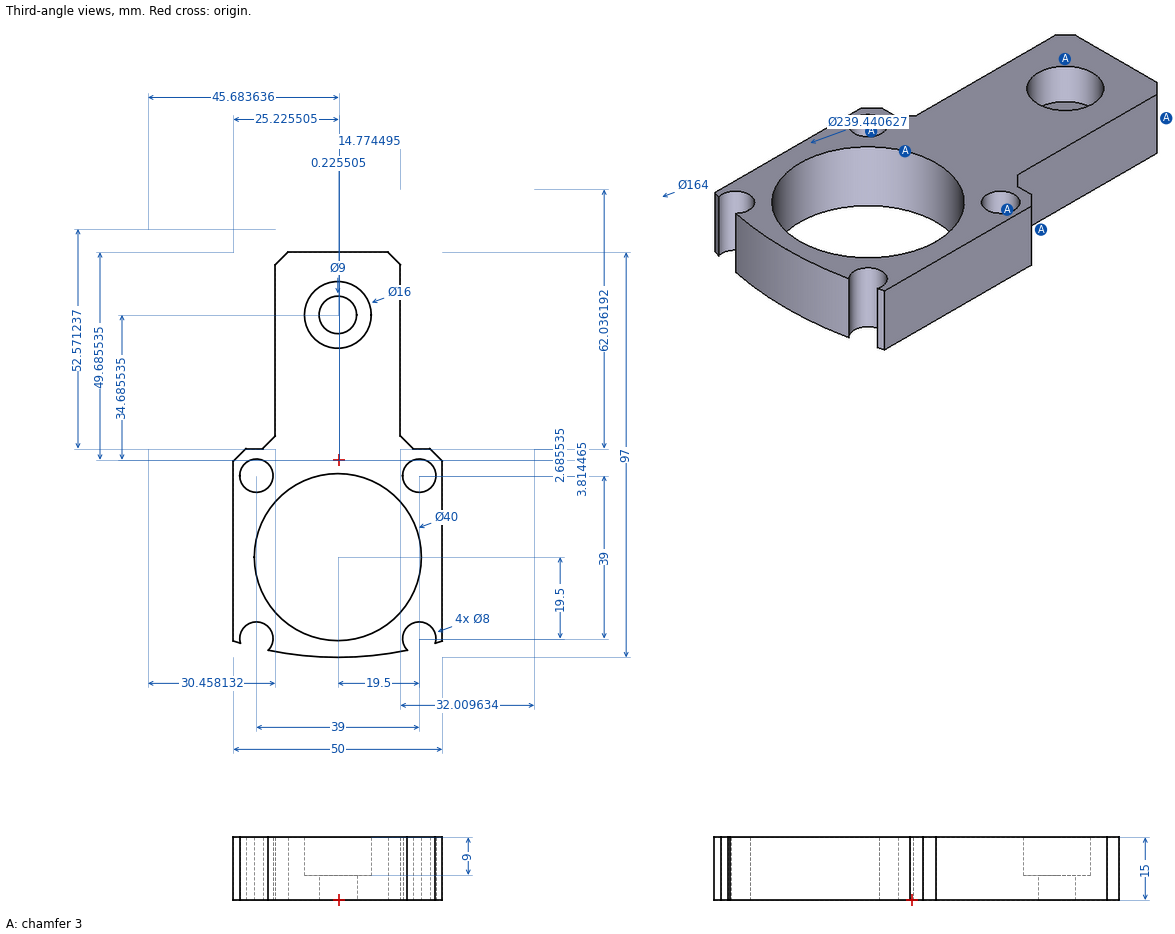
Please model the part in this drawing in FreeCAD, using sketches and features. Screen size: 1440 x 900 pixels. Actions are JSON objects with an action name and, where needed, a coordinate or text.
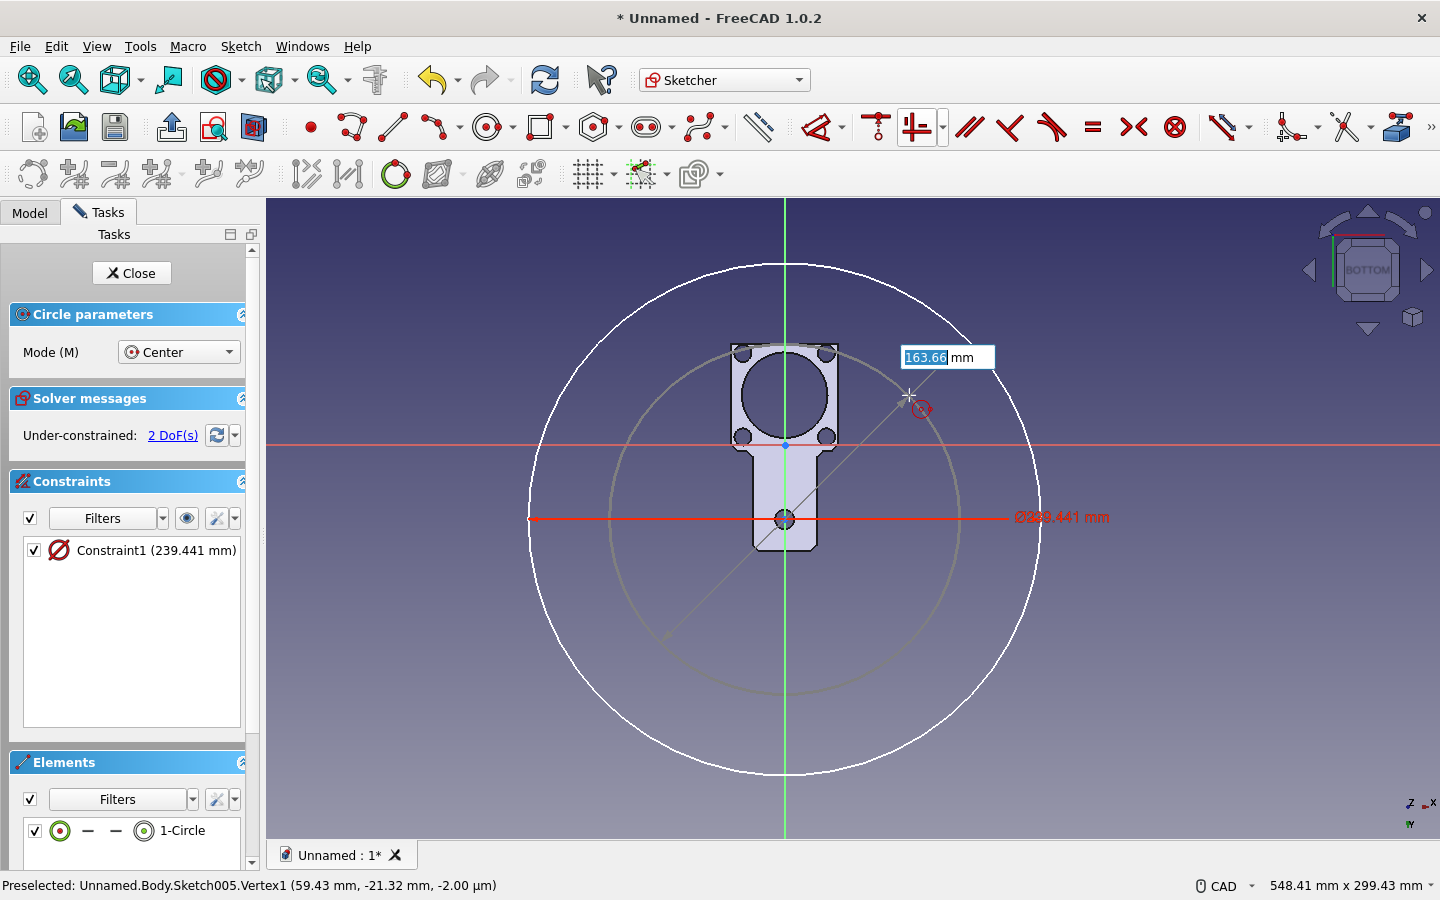
{"action": "type", "text": "164"}
{"action": "key", "text": "Return"}
{"action": "key", "text": "Escape"}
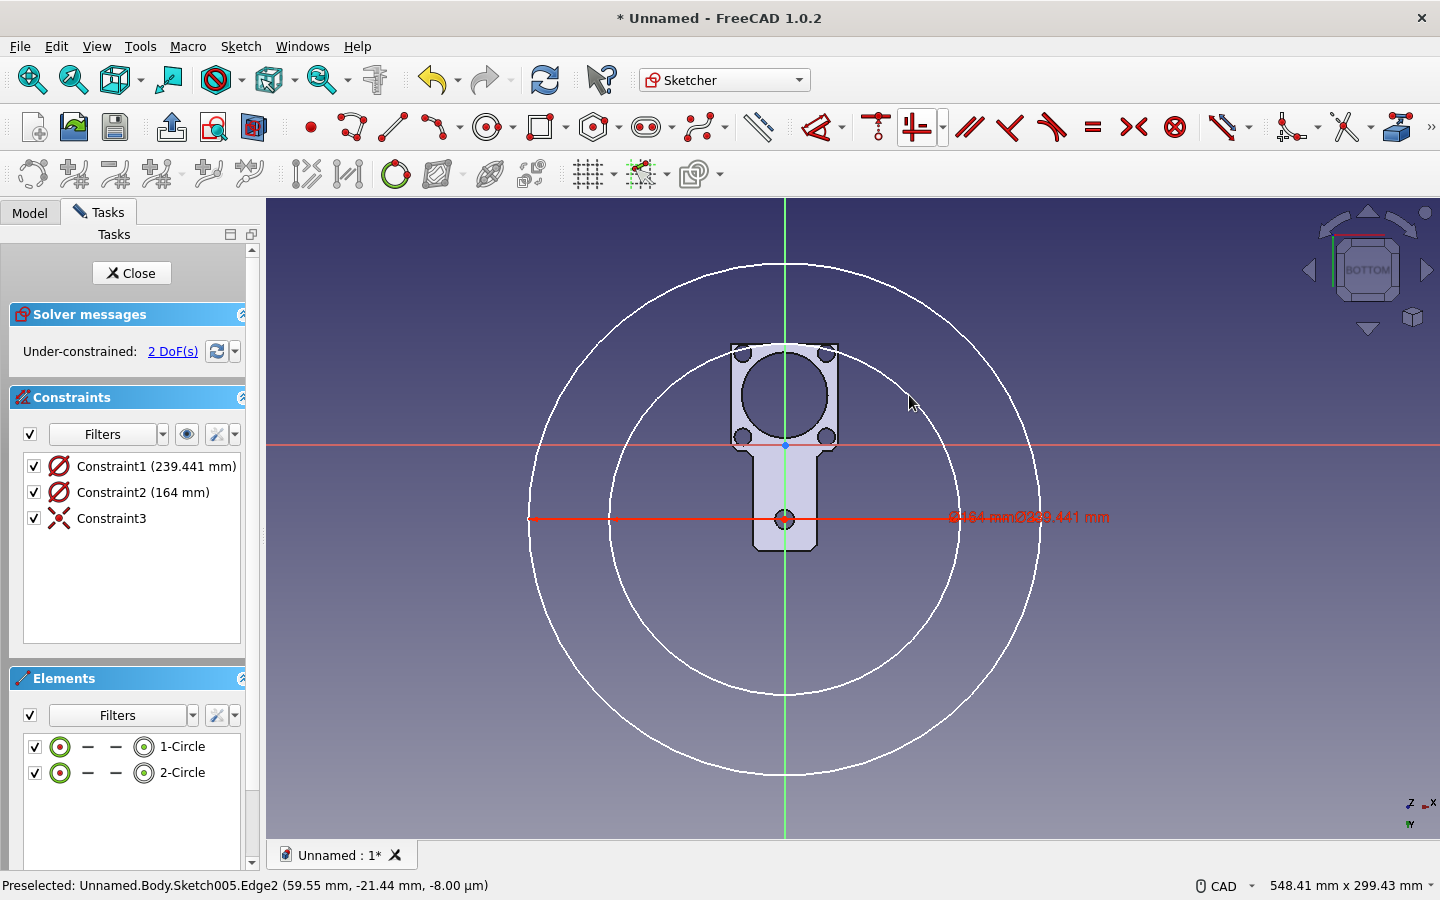
{"action": "key", "text": "d"}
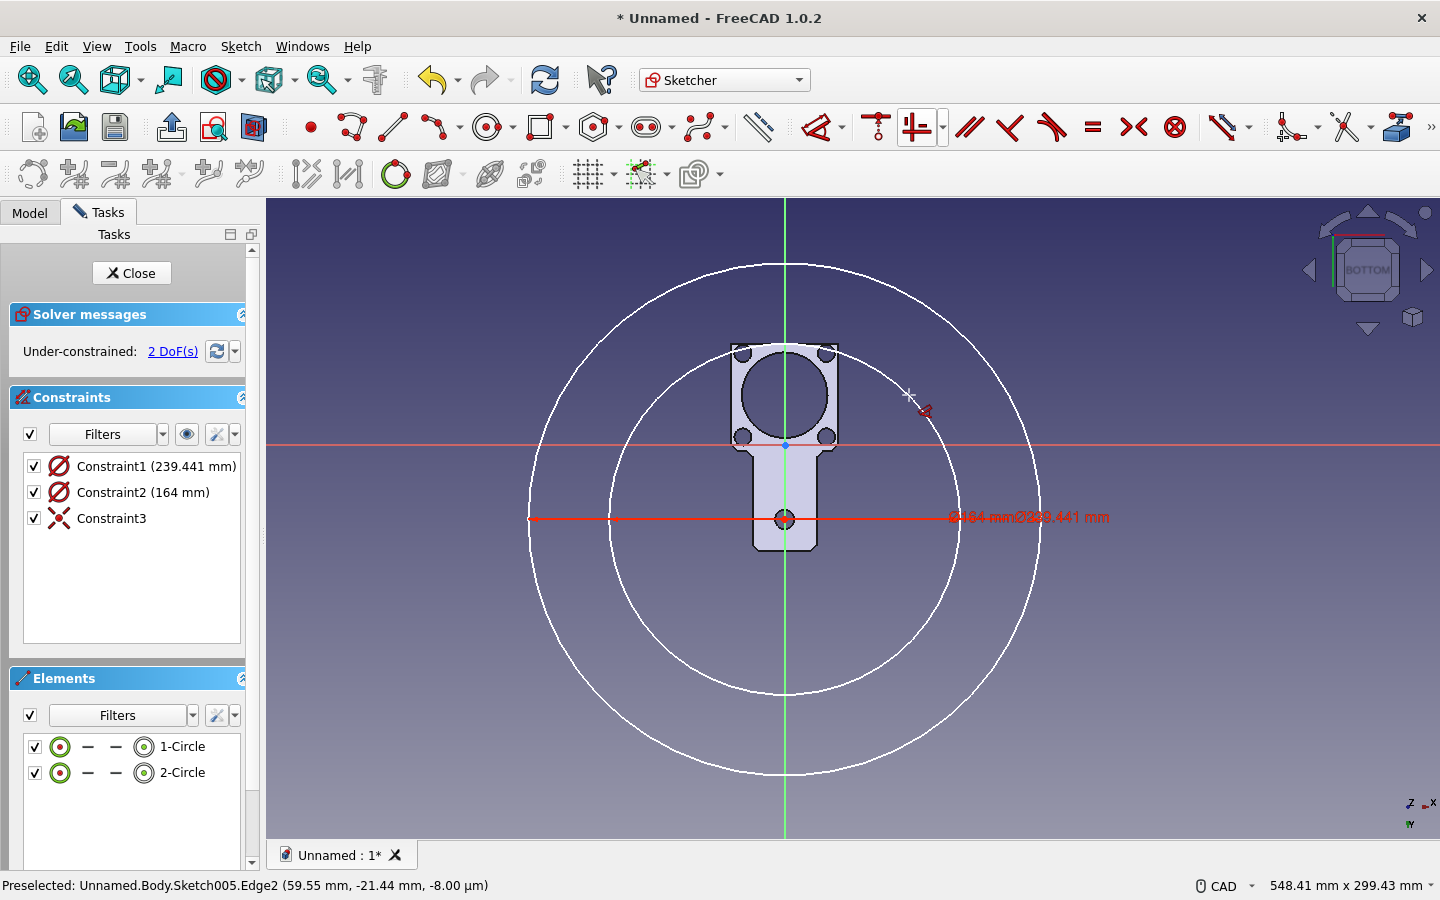
{"action": "scroll", "coordinate": [785, 519], "scroll_direction": "up", "scroll_amount": 23}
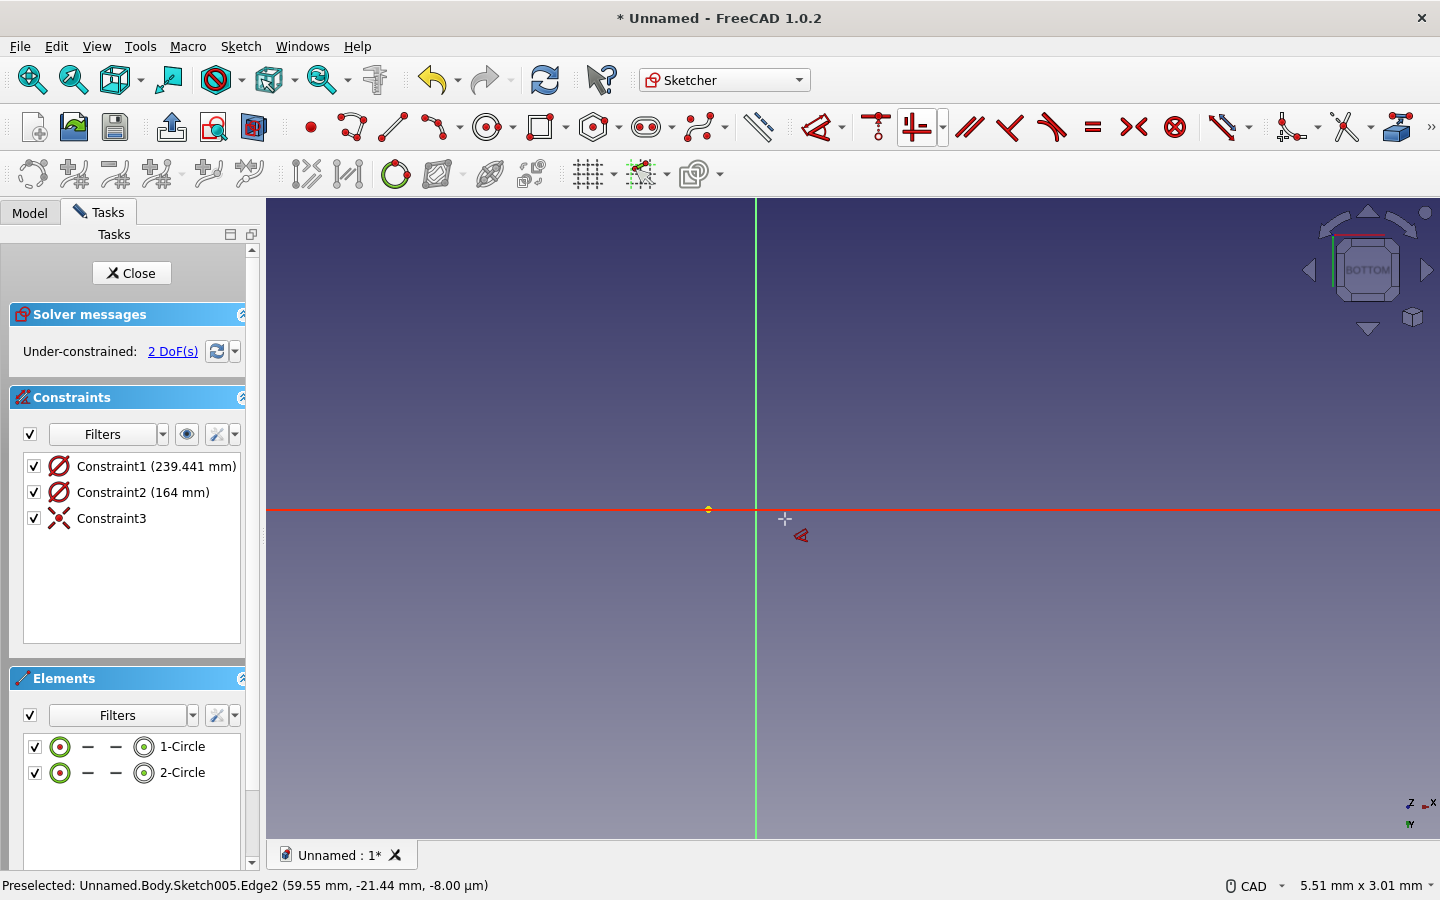
{"action": "left_click", "coordinate": [708, 510]}
{"action": "left_click", "coordinate": [732, 544]}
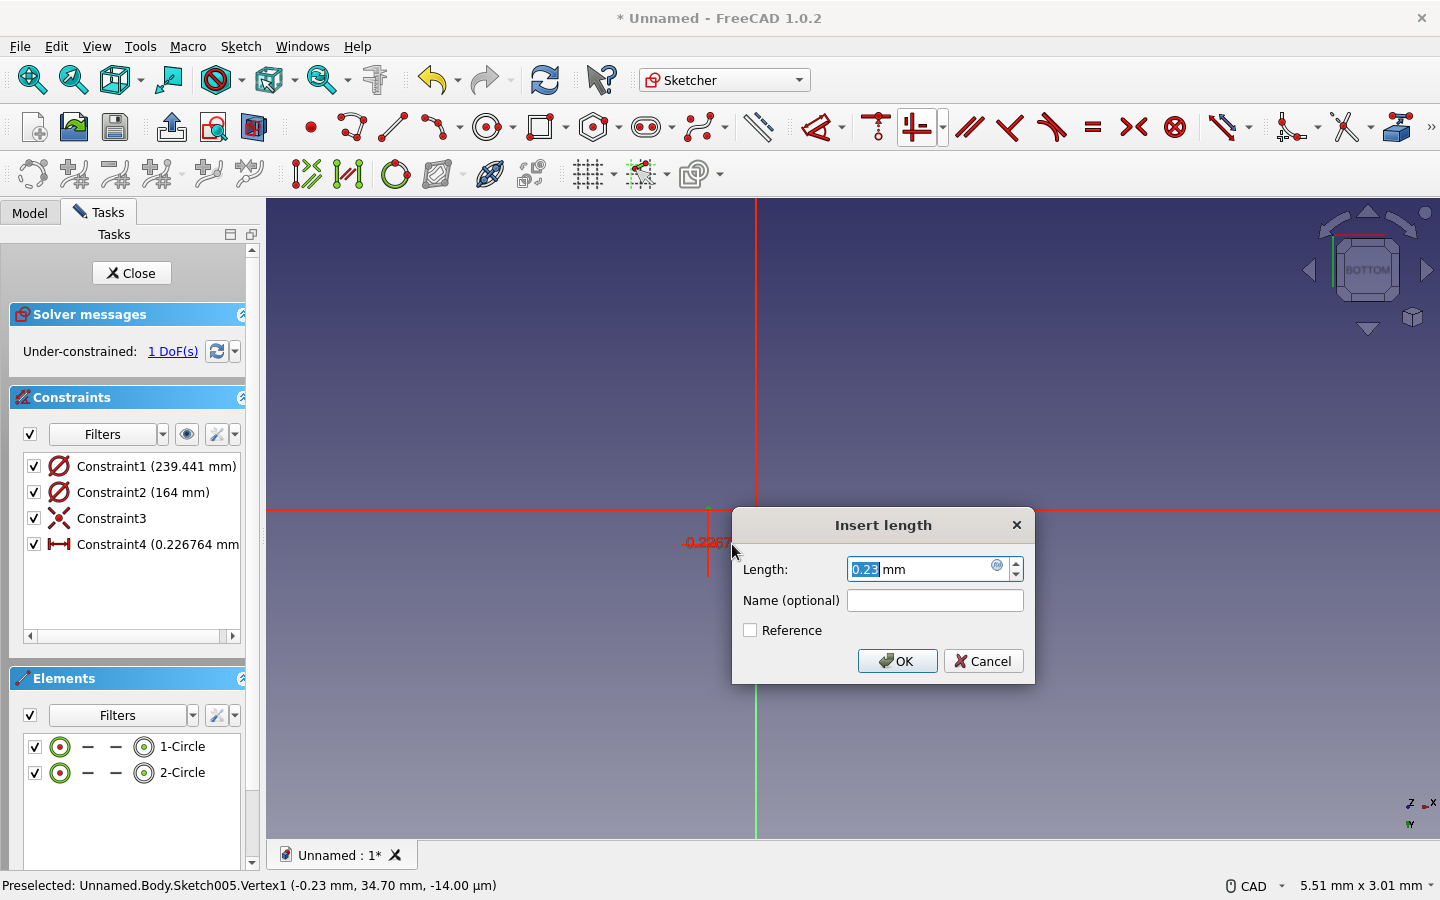
{"action": "type", "text": "0.225505"}
{"action": "key", "text": "Return"}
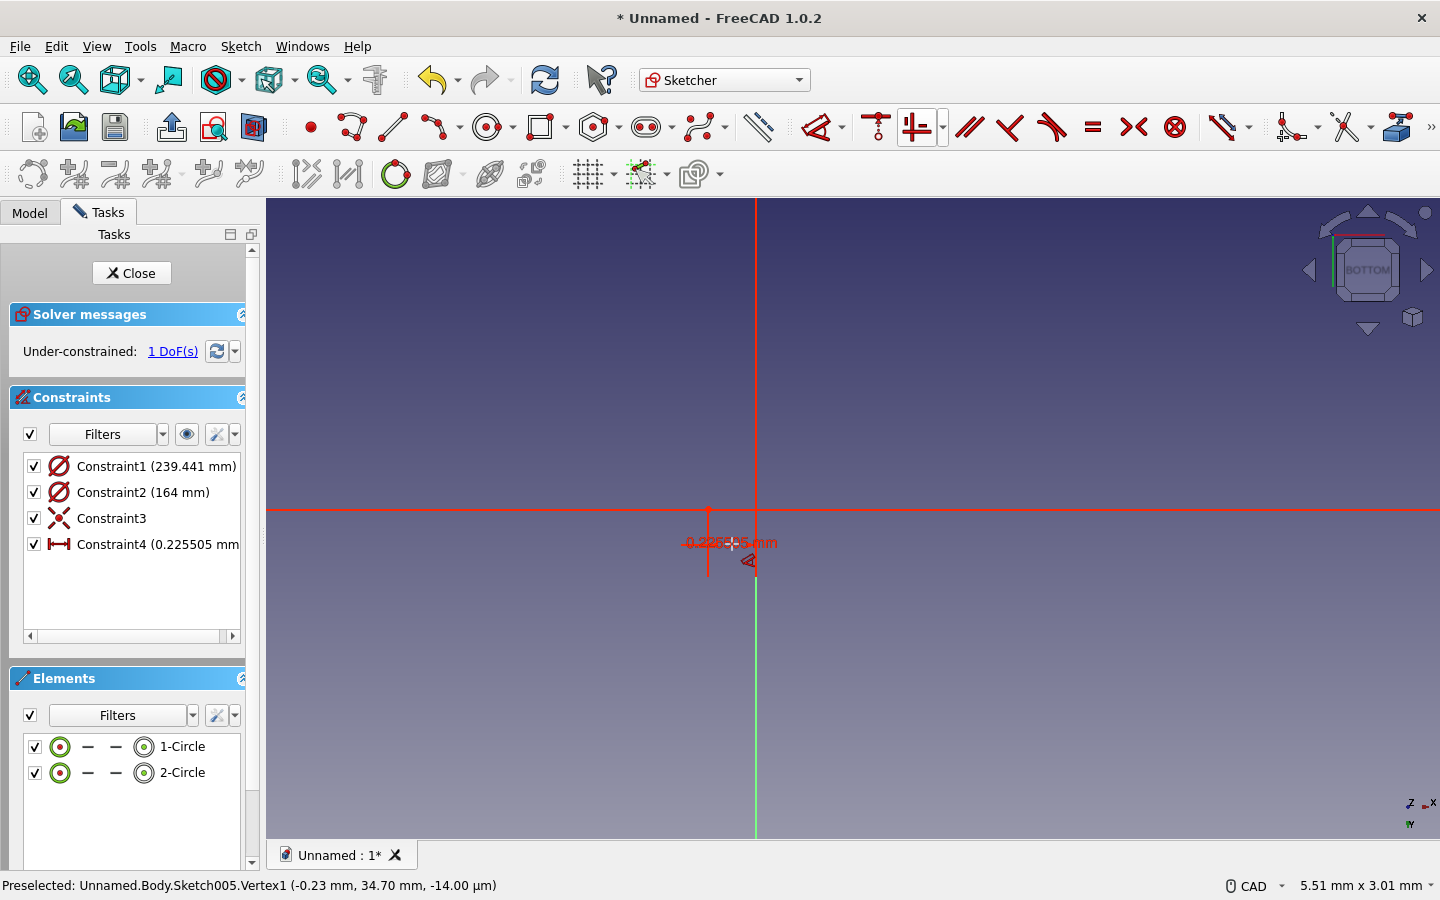
{"action": "scroll", "coordinate": [784, 518], "scroll_direction": "down", "scroll_amount": 15}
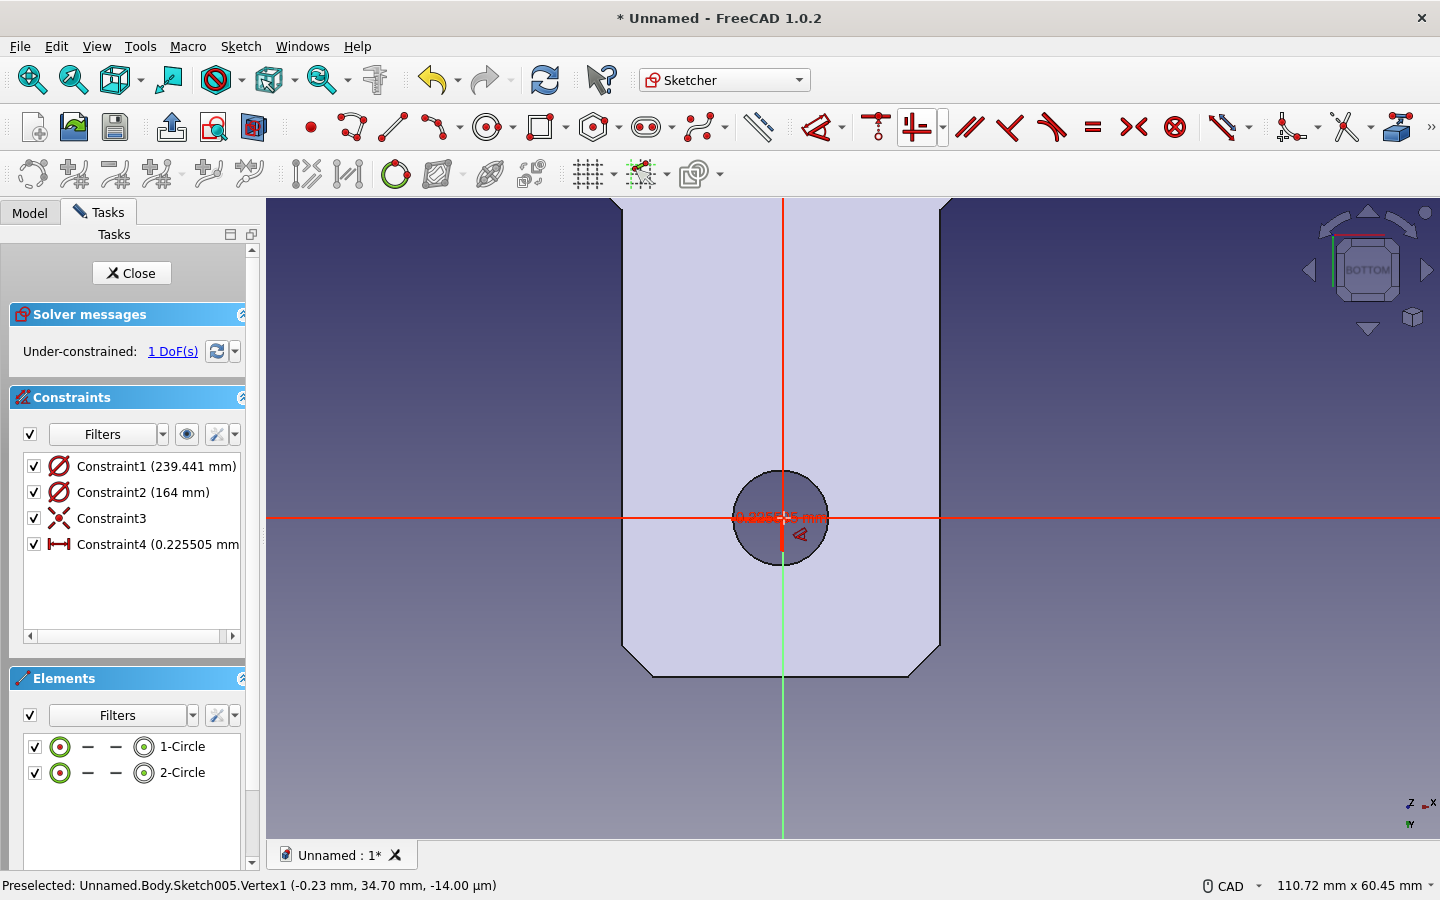
{"action": "scroll", "coordinate": [785, 519], "scroll_direction": "down", "scroll_amount": 9}